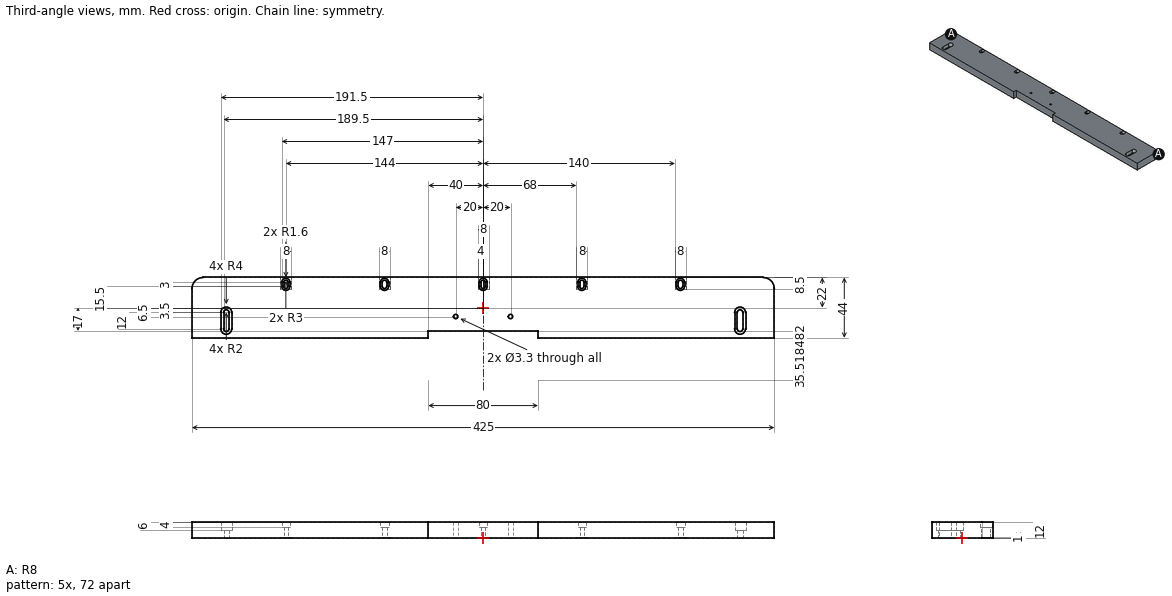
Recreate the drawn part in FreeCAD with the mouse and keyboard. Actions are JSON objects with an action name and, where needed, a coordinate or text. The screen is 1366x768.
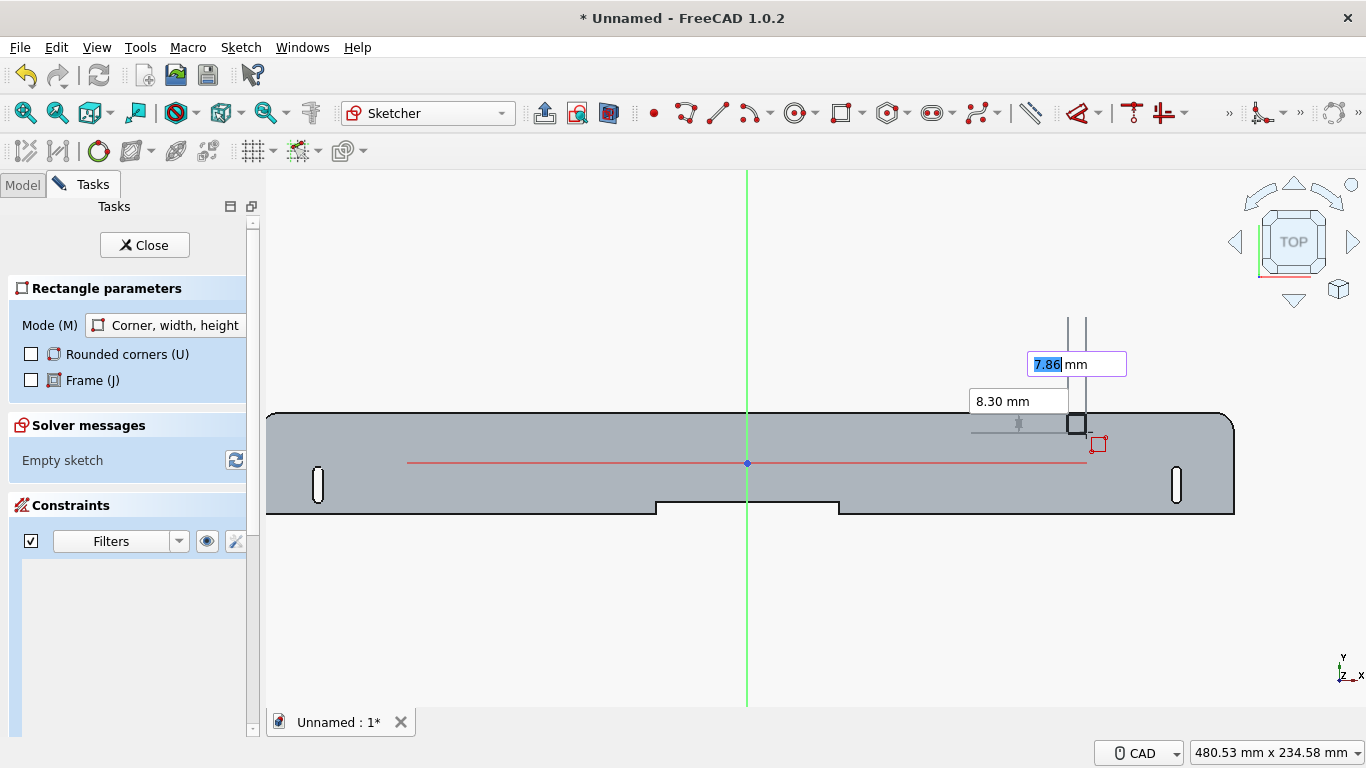
{"action": "type", "text": "8"}
{"action": "key", "text": "Tab"}
{"action": "type", "text": "8.5"}
{"action": "key", "text": "Return"}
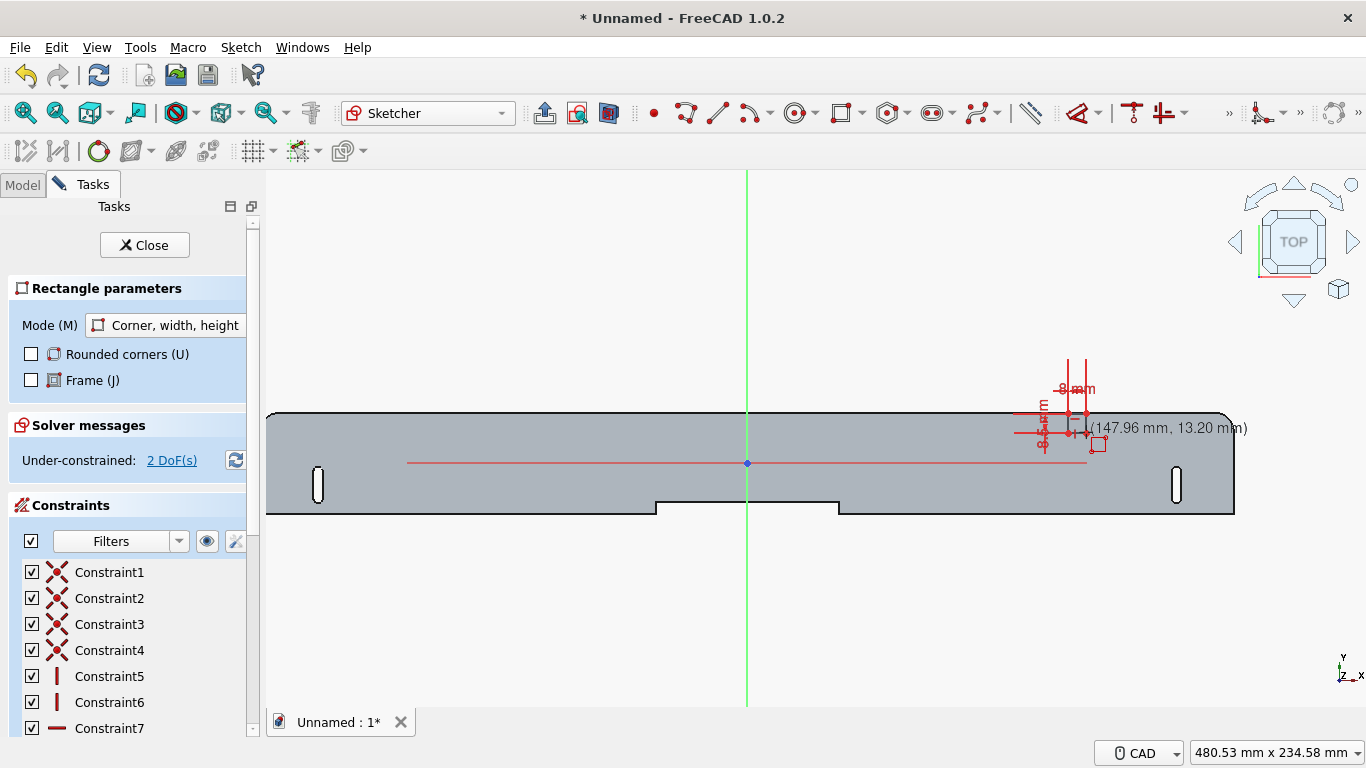
{"action": "left_click", "coordinate": [903, 413]}
{"action": "mouse_move", "coordinate": [921, 432]}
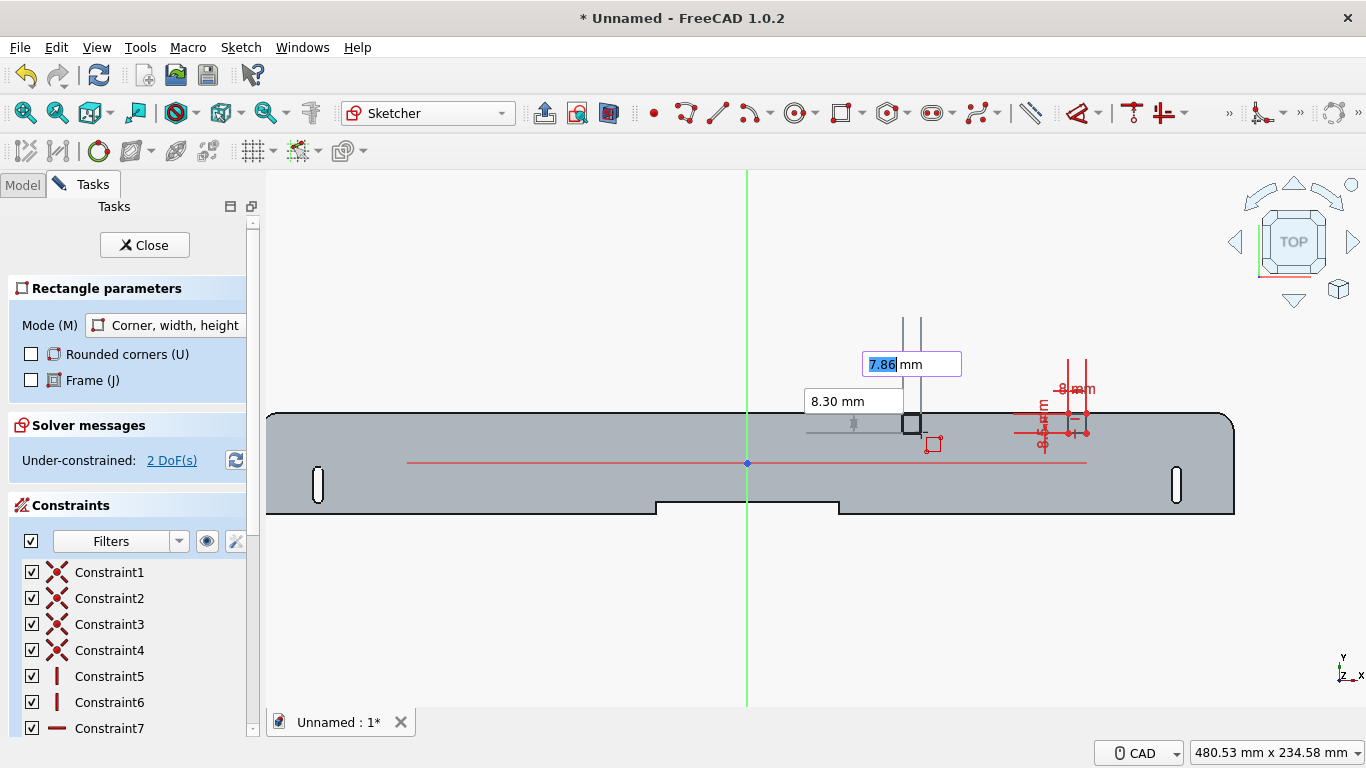
{"action": "type", "text": "8"}
{"action": "key", "text": "Tab"}
{"action": "type", "text": "8.5"}
{"action": "key", "text": "Return"}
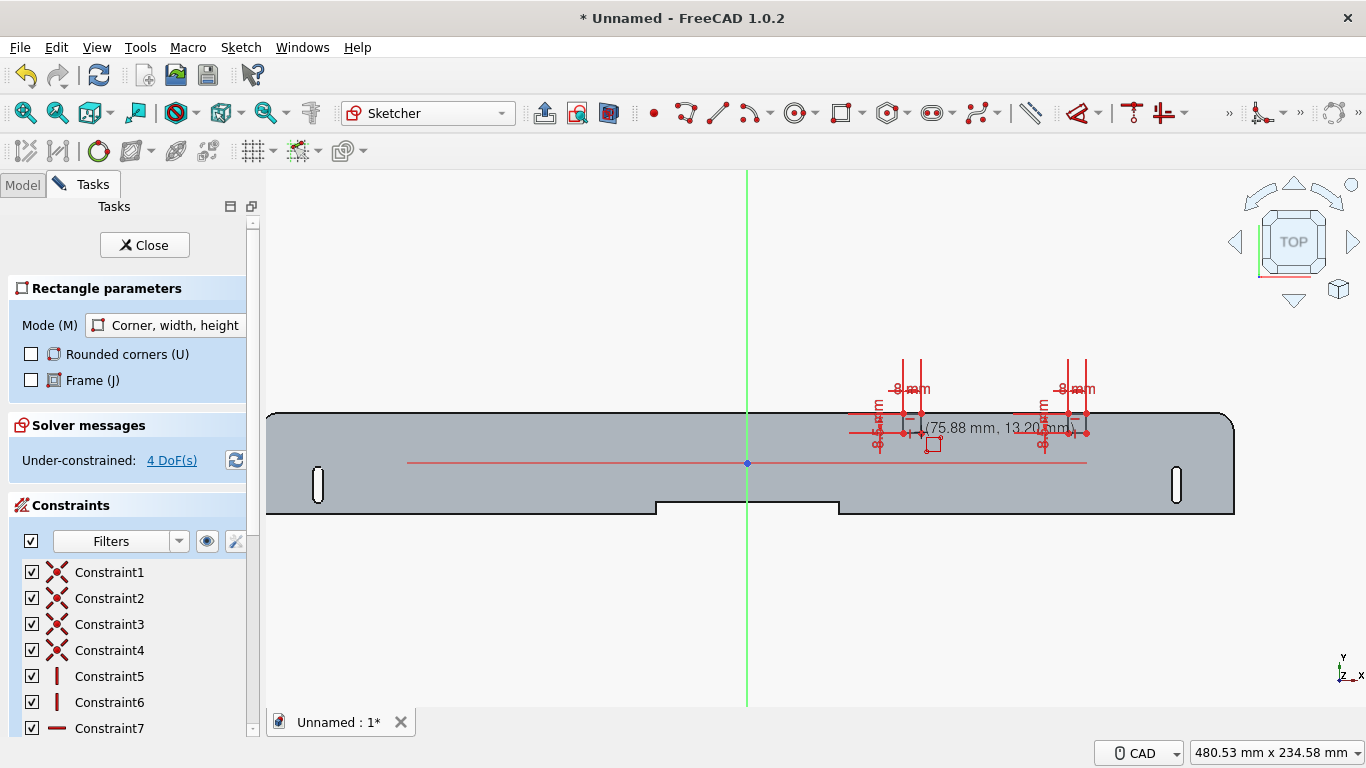
{"action": "scroll", "coordinate": [738, 413], "scroll_direction": "up", "scroll_amount": 3}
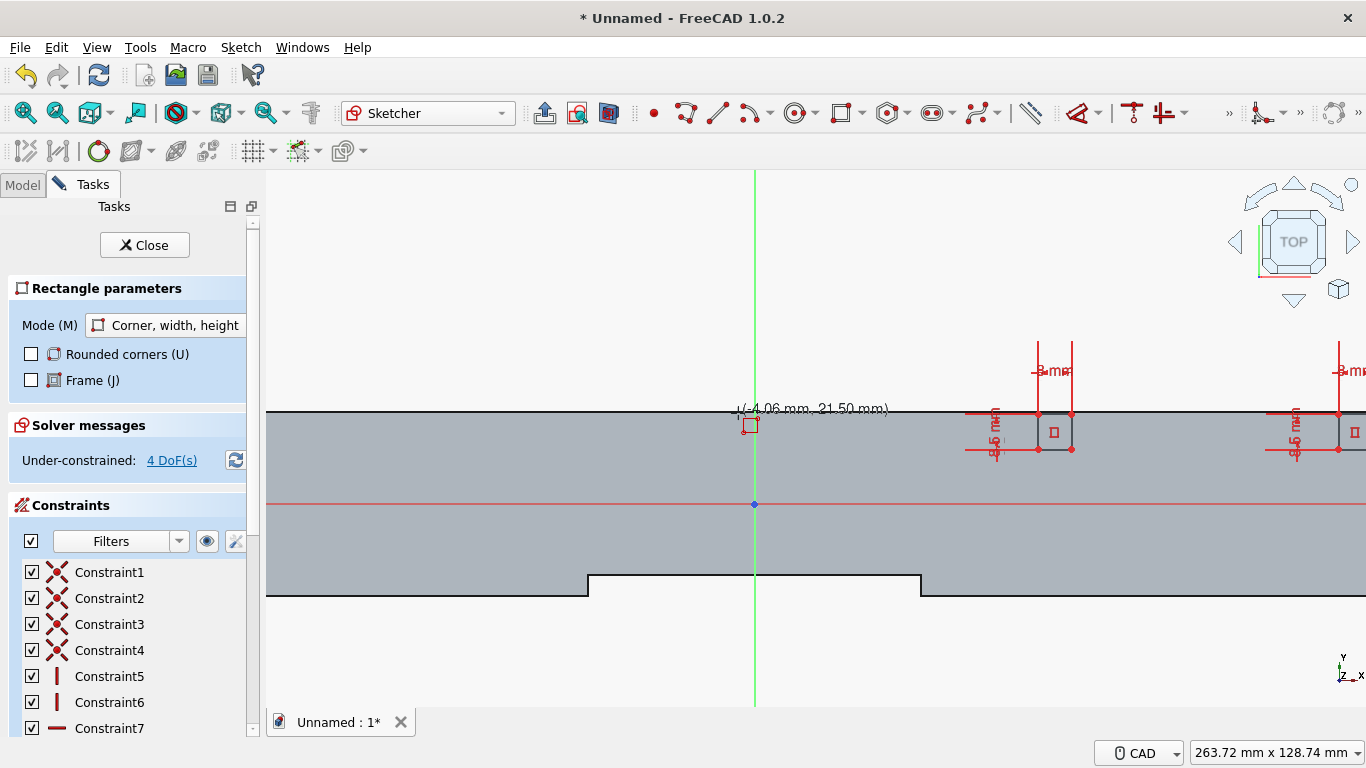
{"action": "left_click", "coordinate": [738, 412]}
{"action": "mouse_move", "coordinate": [771, 448]}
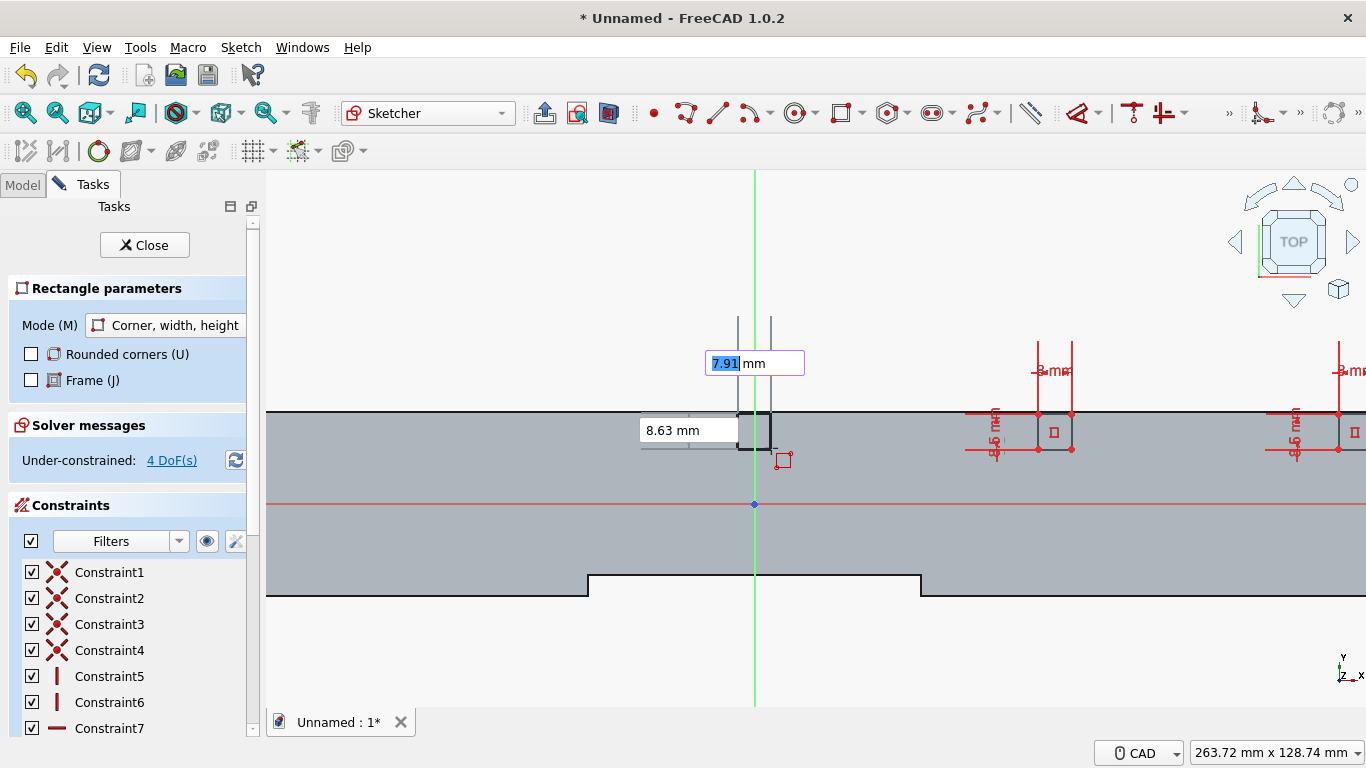
{"action": "type", "text": "8"}
{"action": "key", "text": "Tab"}
{"action": "type", "text": "8.5"}
{"action": "key", "text": "Return"}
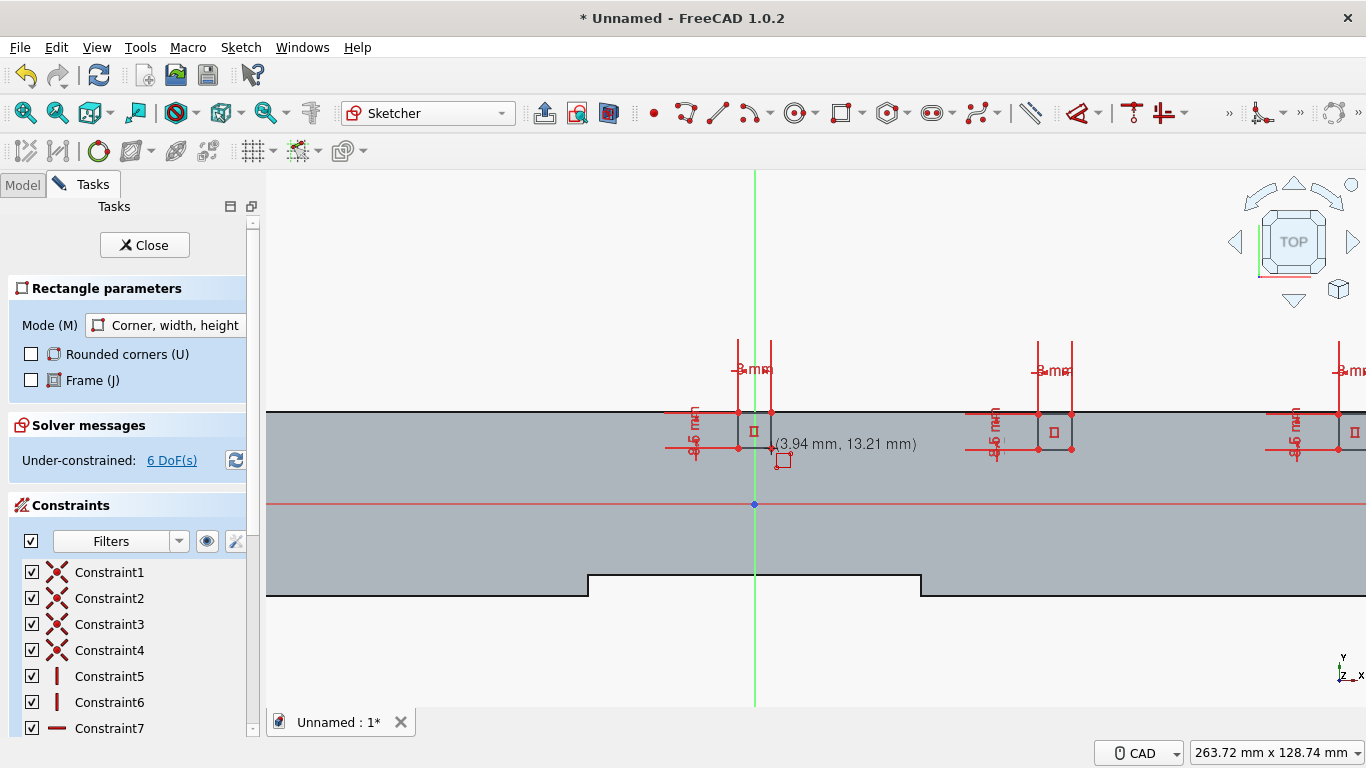
{"action": "left_click", "coordinate": [438, 412]}
{"action": "mouse_move", "coordinate": [471, 448]}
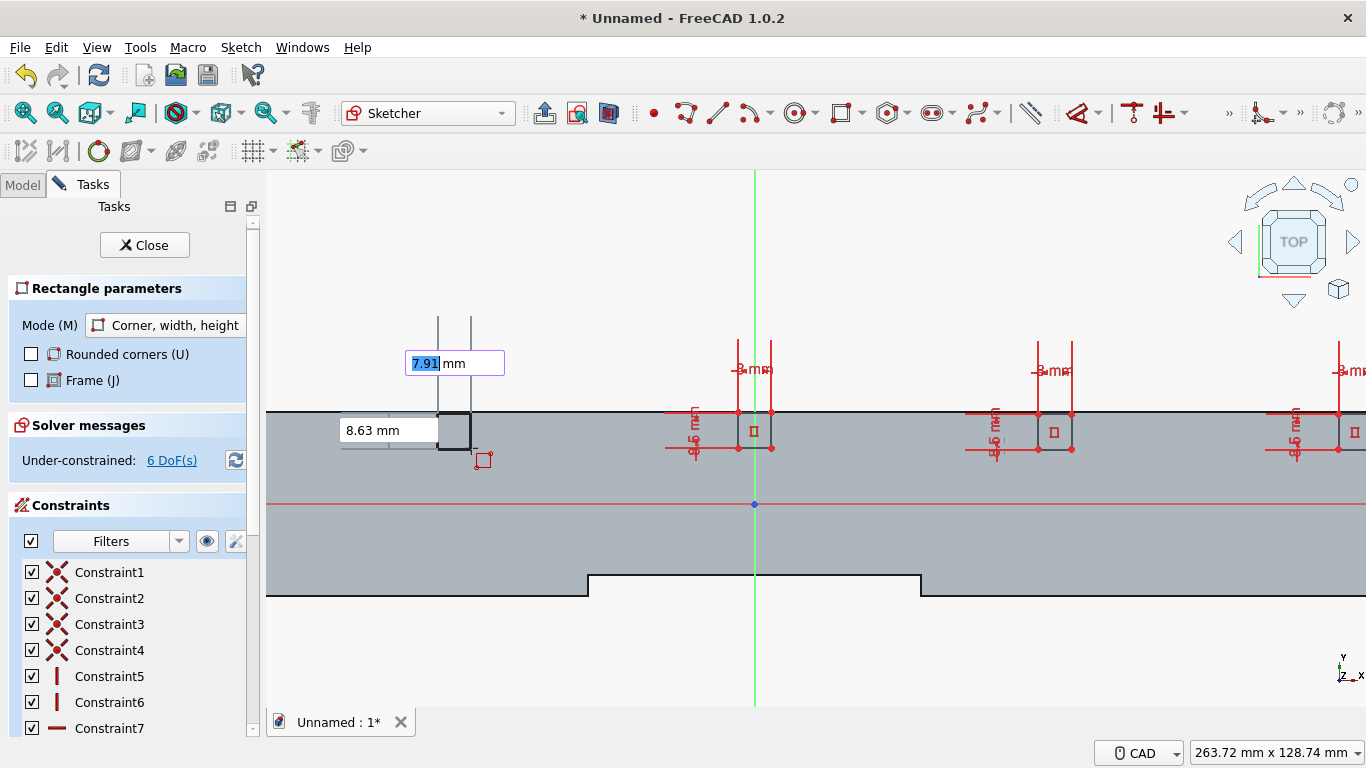
{"action": "type", "text": "8"}
{"action": "key", "text": "Tab"}
{"action": "type", "text": "8.5"}
{"action": "key", "text": "Return"}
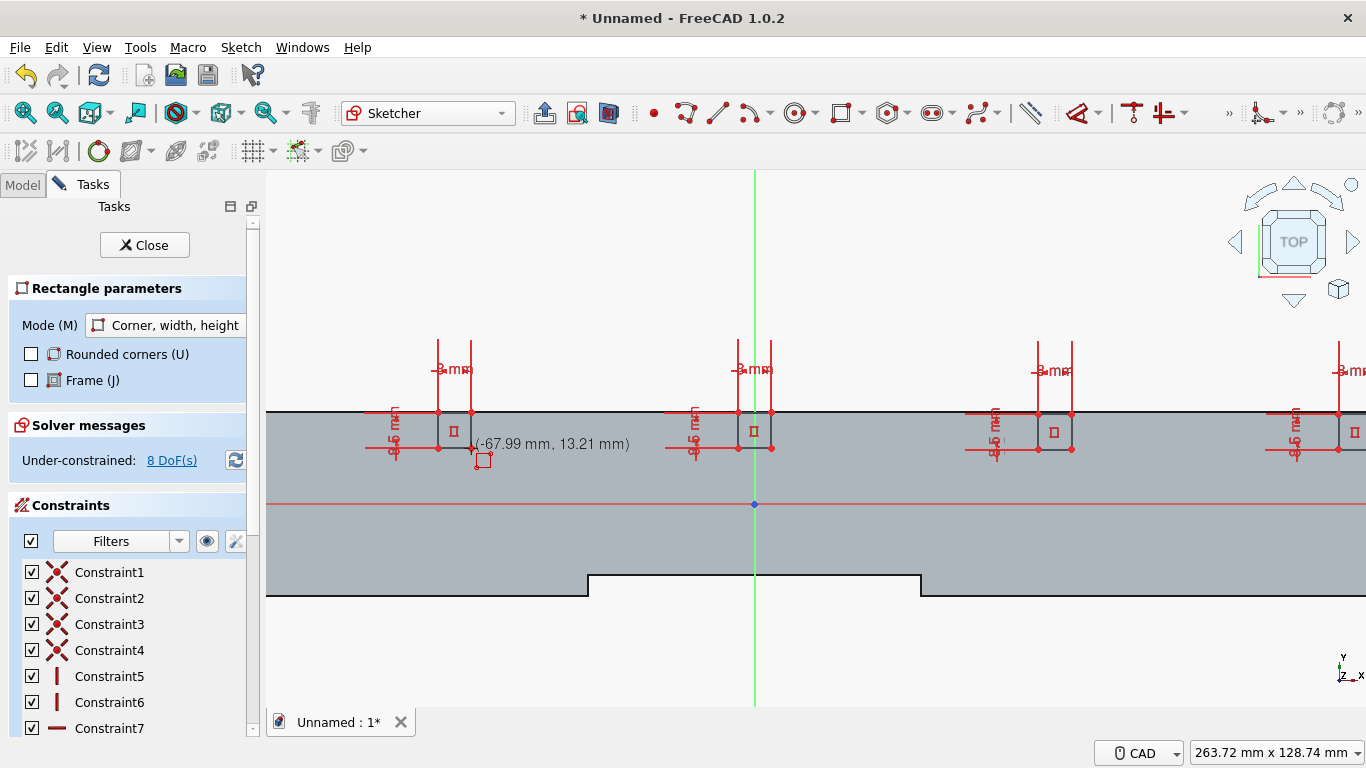
{"action": "scroll", "coordinate": [739, 414], "scroll_direction": "down", "scroll_amount": 3}